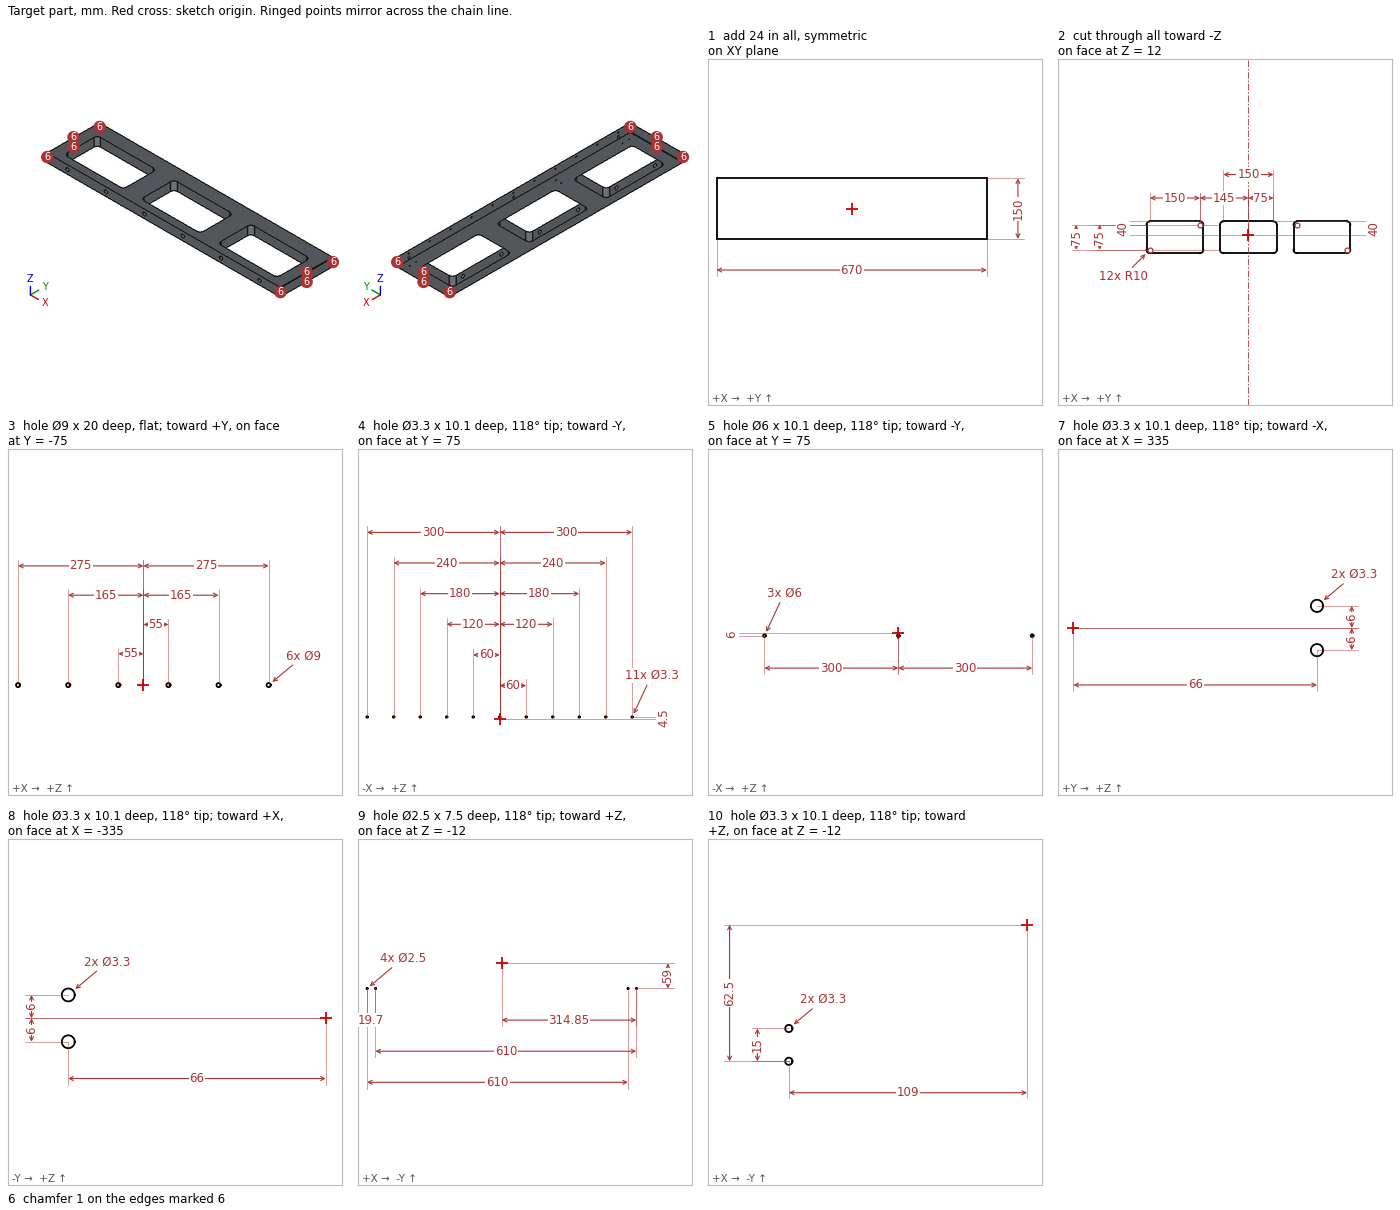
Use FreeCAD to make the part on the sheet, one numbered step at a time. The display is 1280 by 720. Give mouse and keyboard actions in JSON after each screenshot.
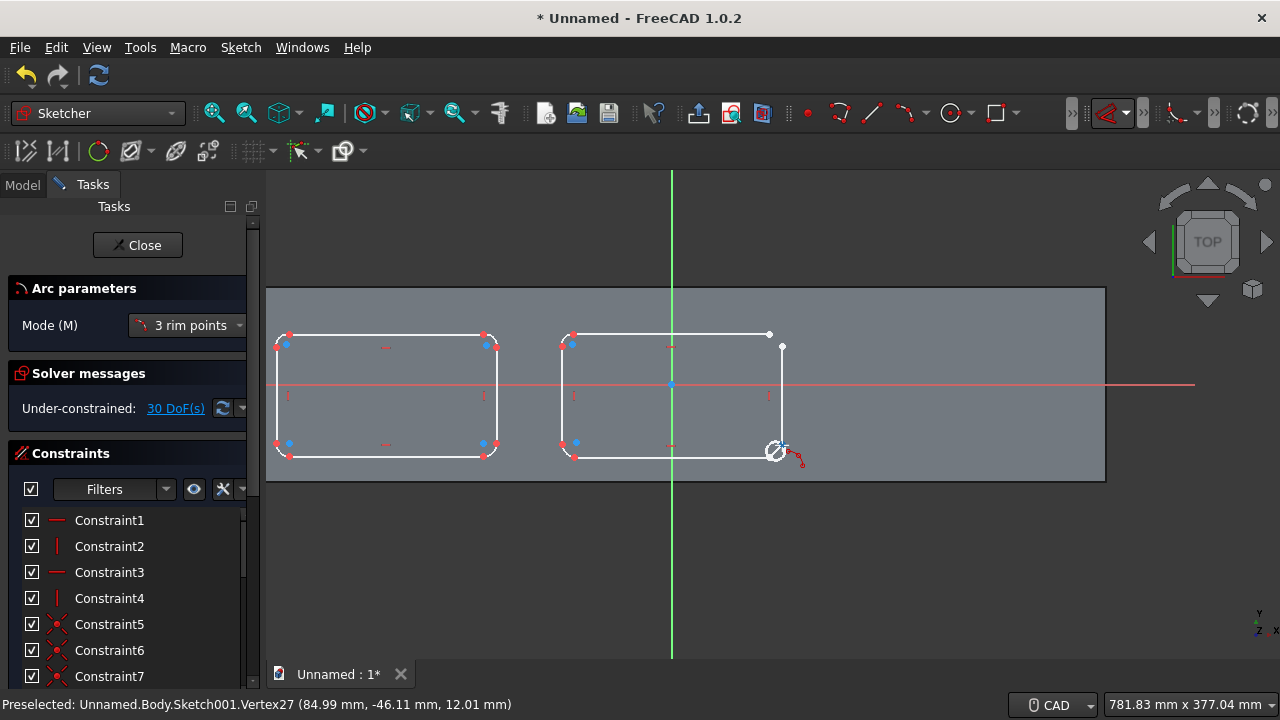
{"action": "scroll", "coordinate": [778, 452], "scroll_direction": "up", "scroll_amount": 8}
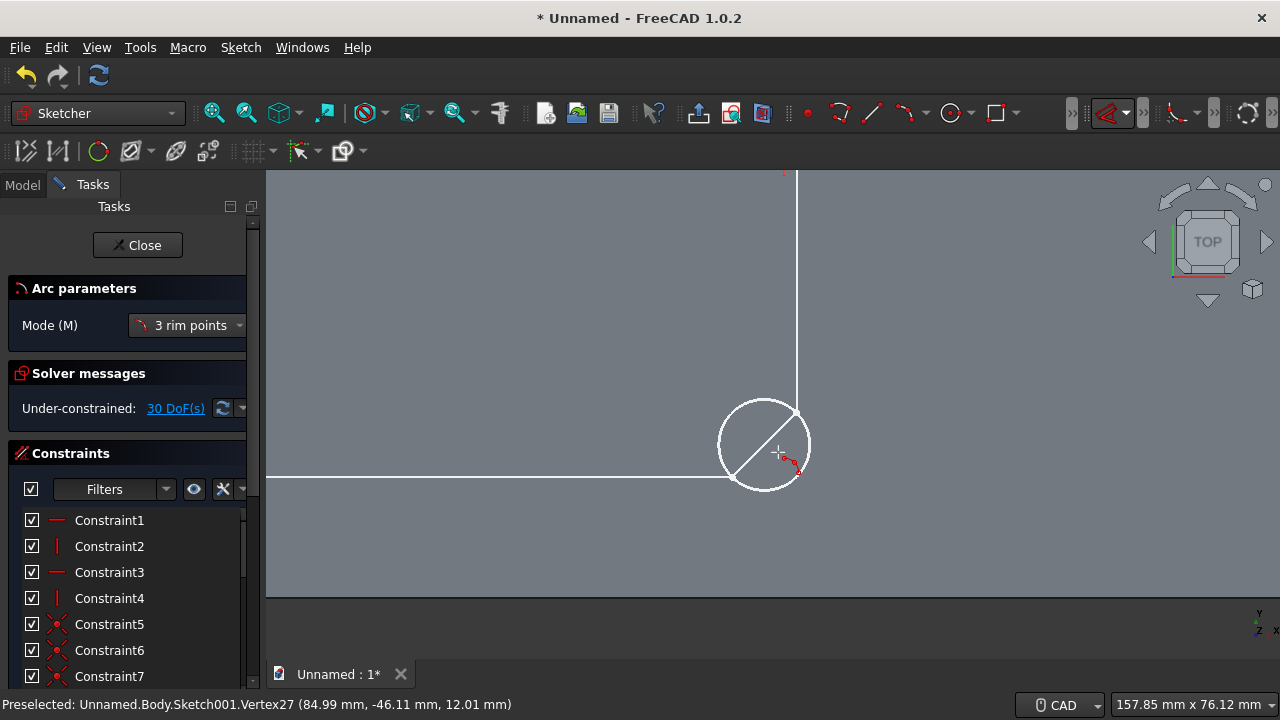
{"action": "left_click", "coordinate": [778, 451]}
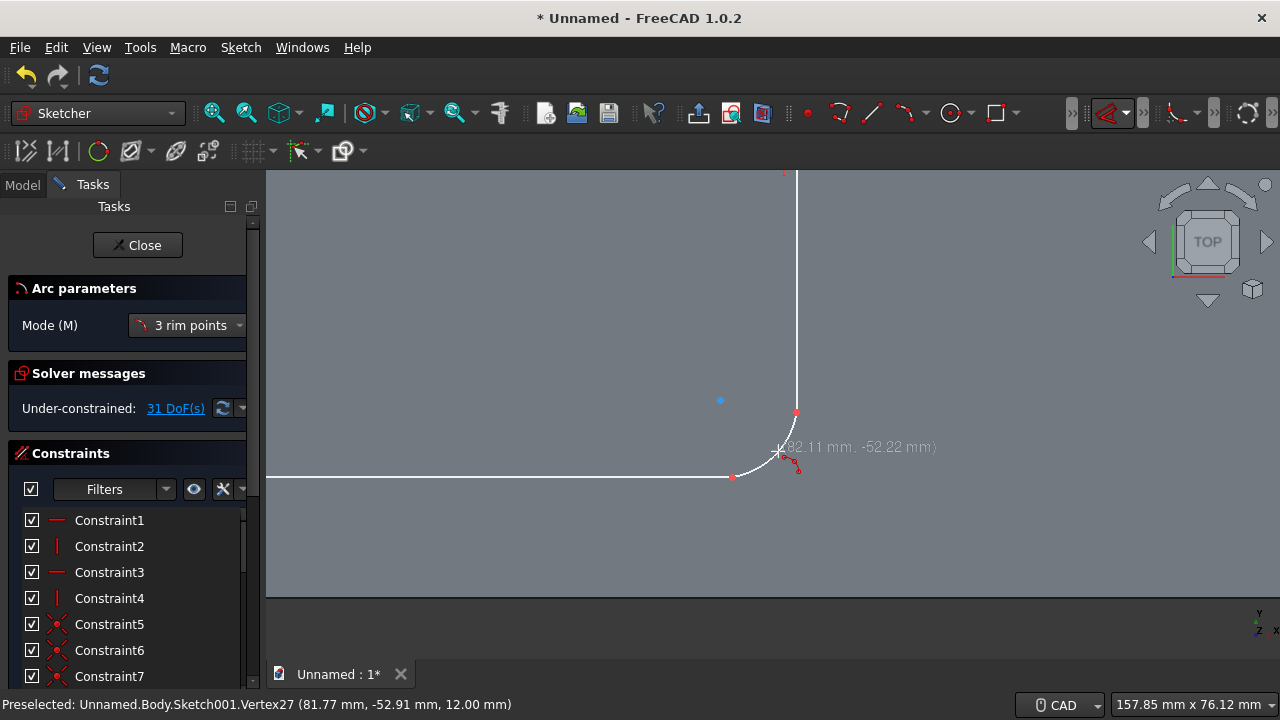
{"action": "scroll", "coordinate": [776, 454], "scroll_direction": "down", "scroll_amount": 10}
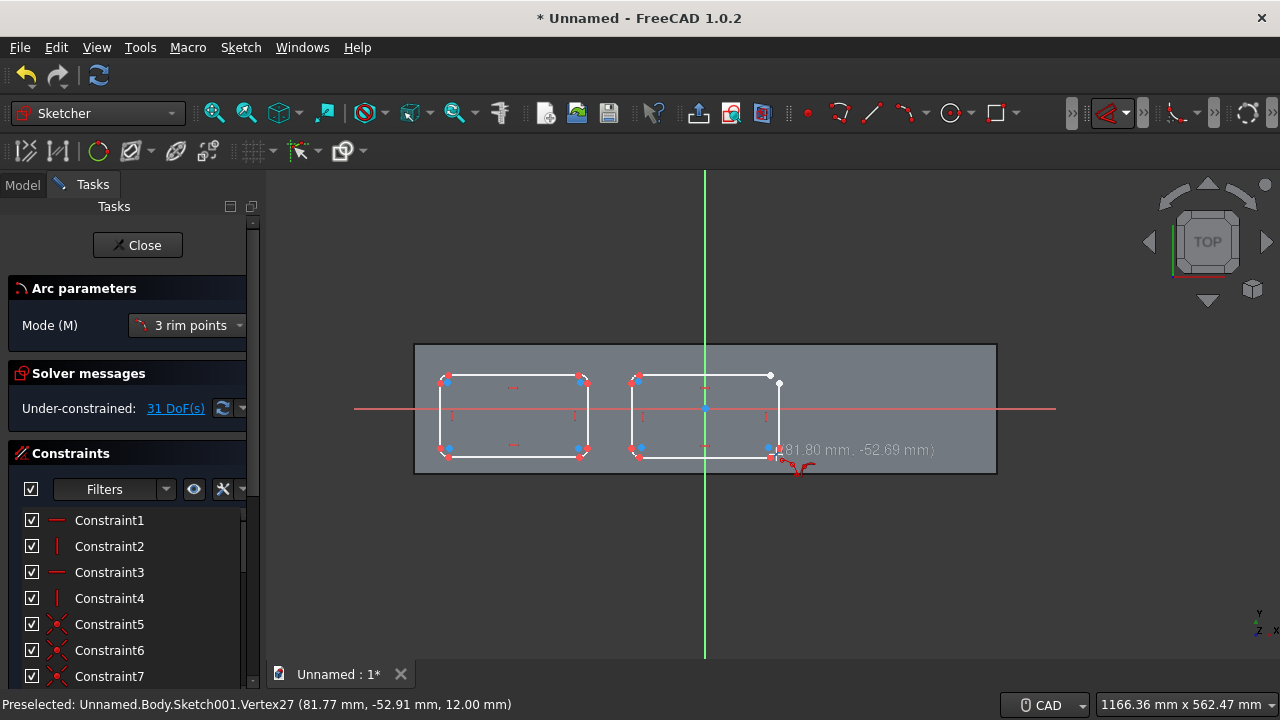
{"action": "scroll", "coordinate": [779, 383], "scroll_direction": "up", "scroll_amount": 2}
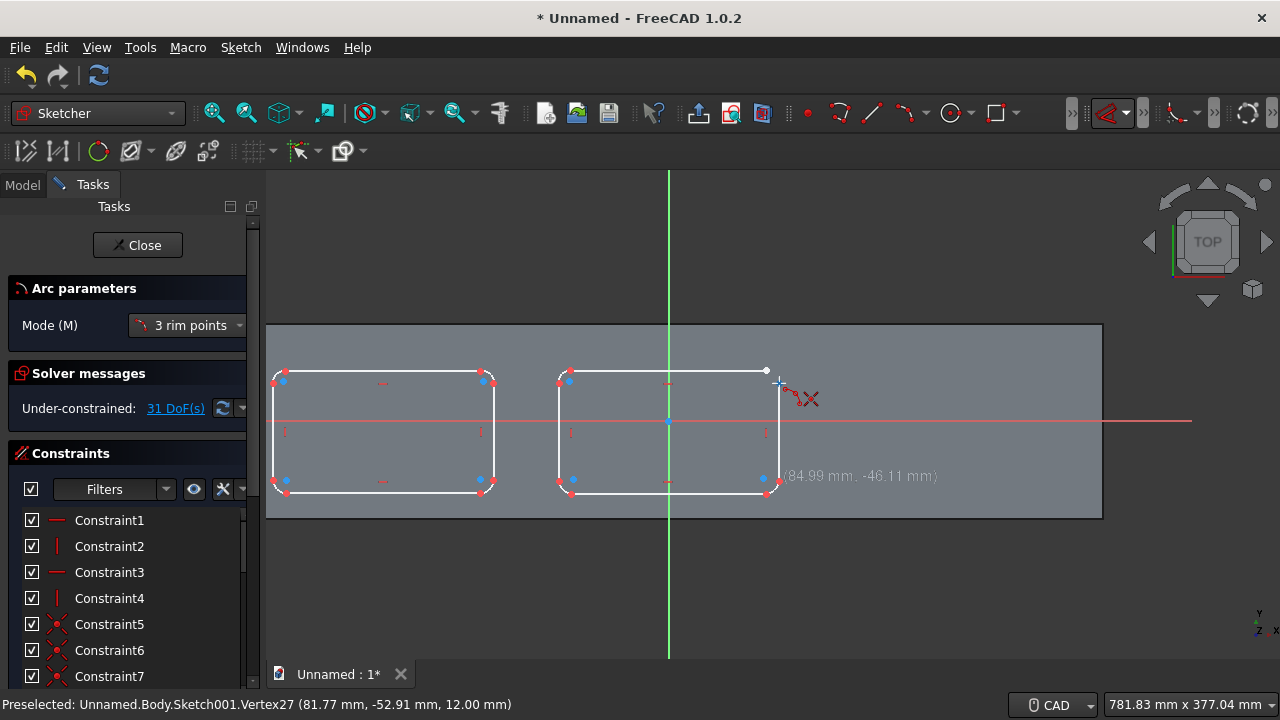
{"action": "left_click", "coordinate": [779, 383]}
{"action": "left_click", "coordinate": [766, 371]}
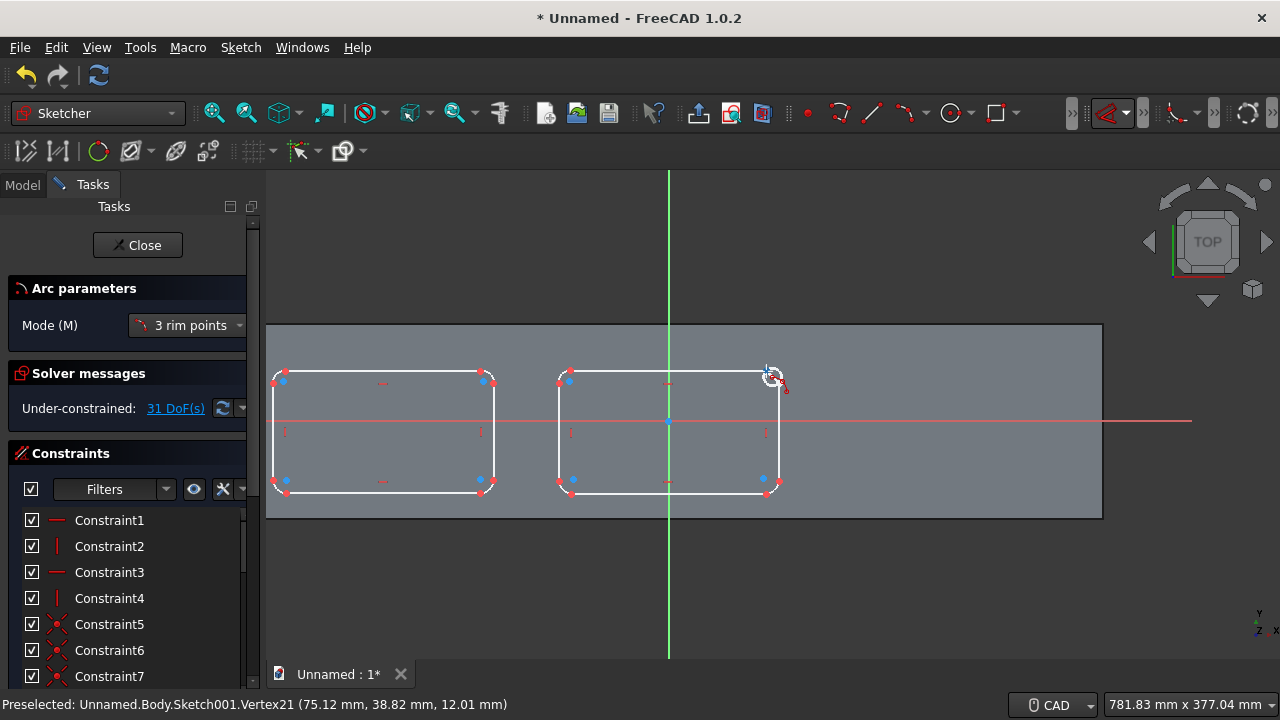
{"action": "scroll", "coordinate": [775, 373], "scroll_direction": "up", "scroll_amount": 8}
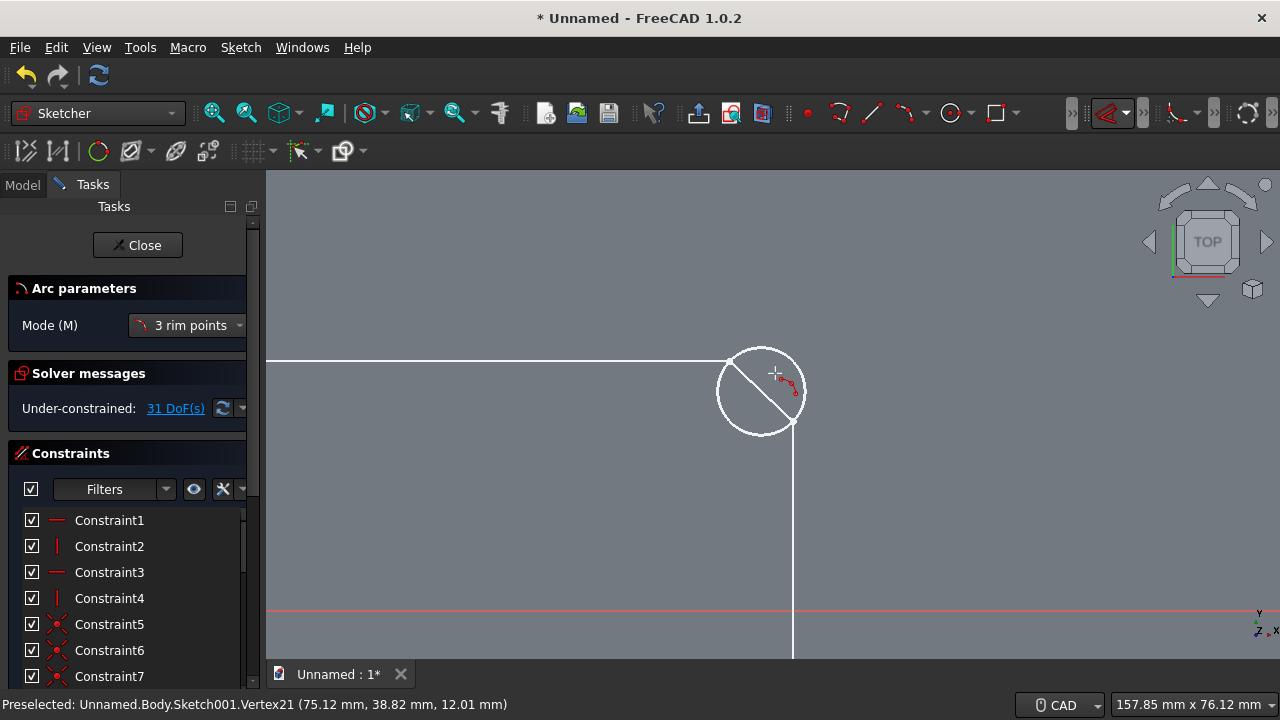
{"action": "left_click", "coordinate": [774, 373]}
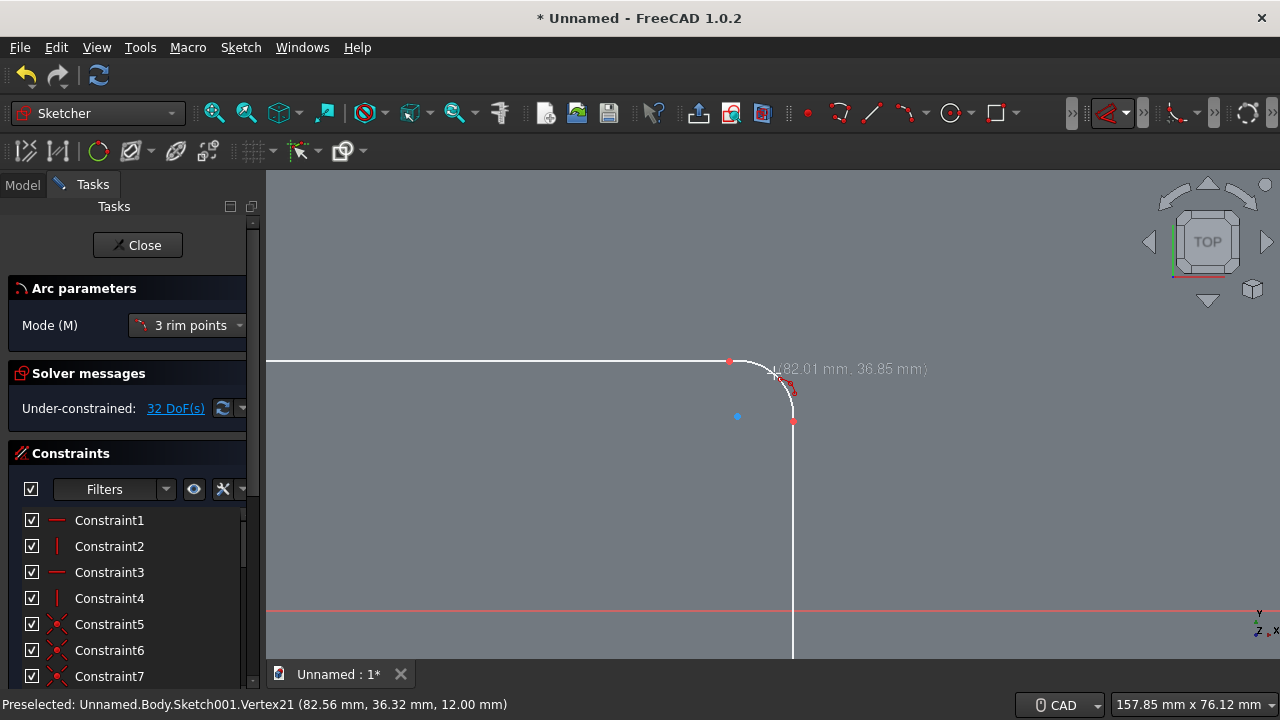
{"action": "left_click", "coordinate": [872, 114]}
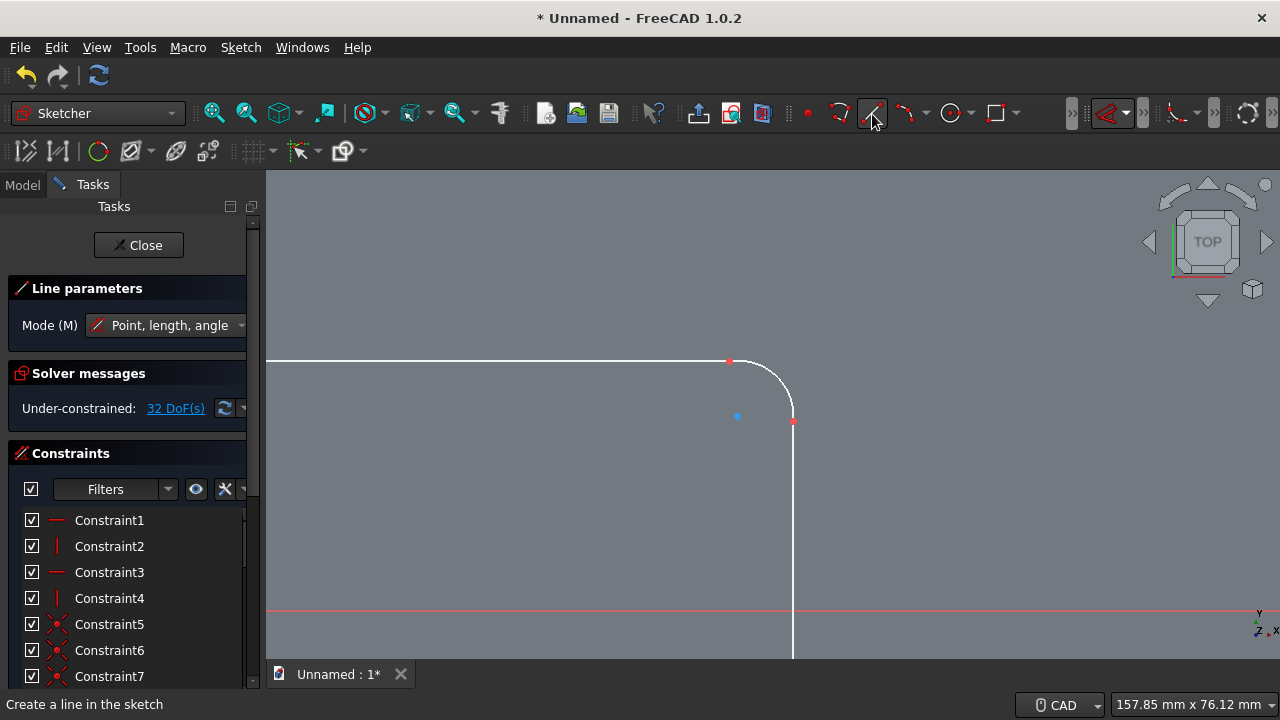
{"action": "scroll", "coordinate": [776, 376], "scroll_direction": "down", "scroll_amount": 10}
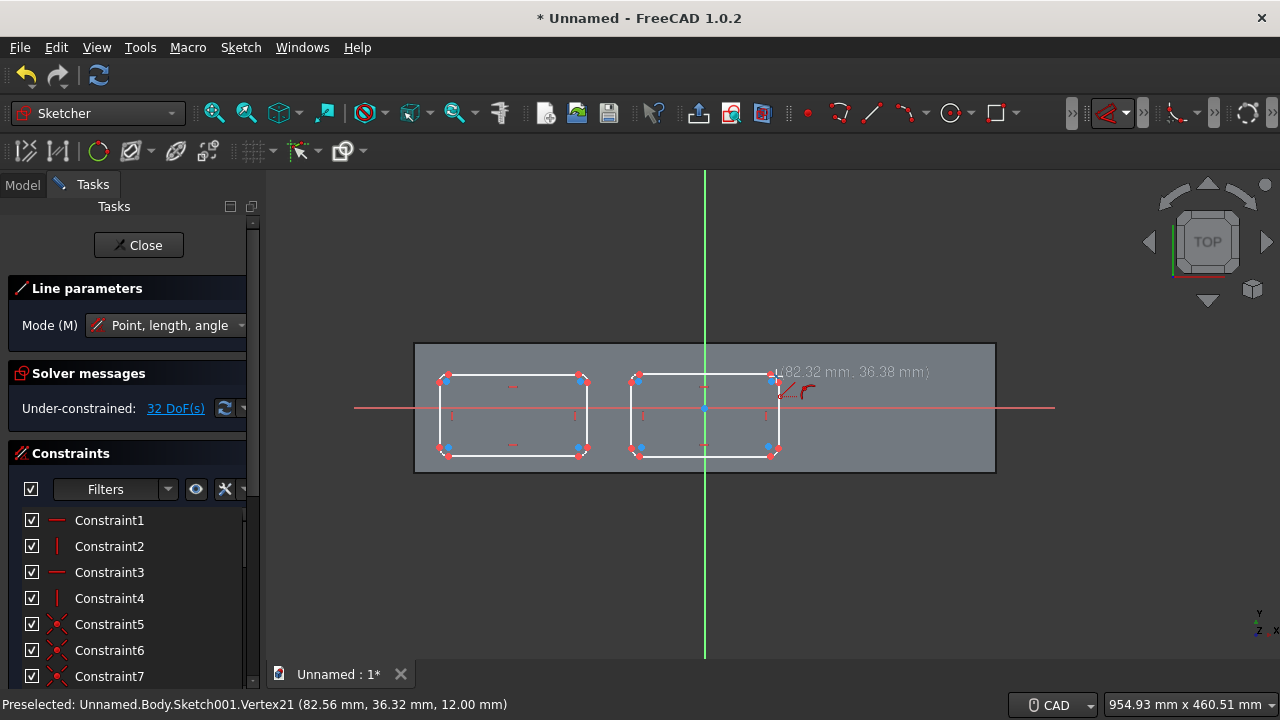
{"action": "left_click", "coordinate": [961, 373]}
{"action": "left_click", "coordinate": [831, 373]}